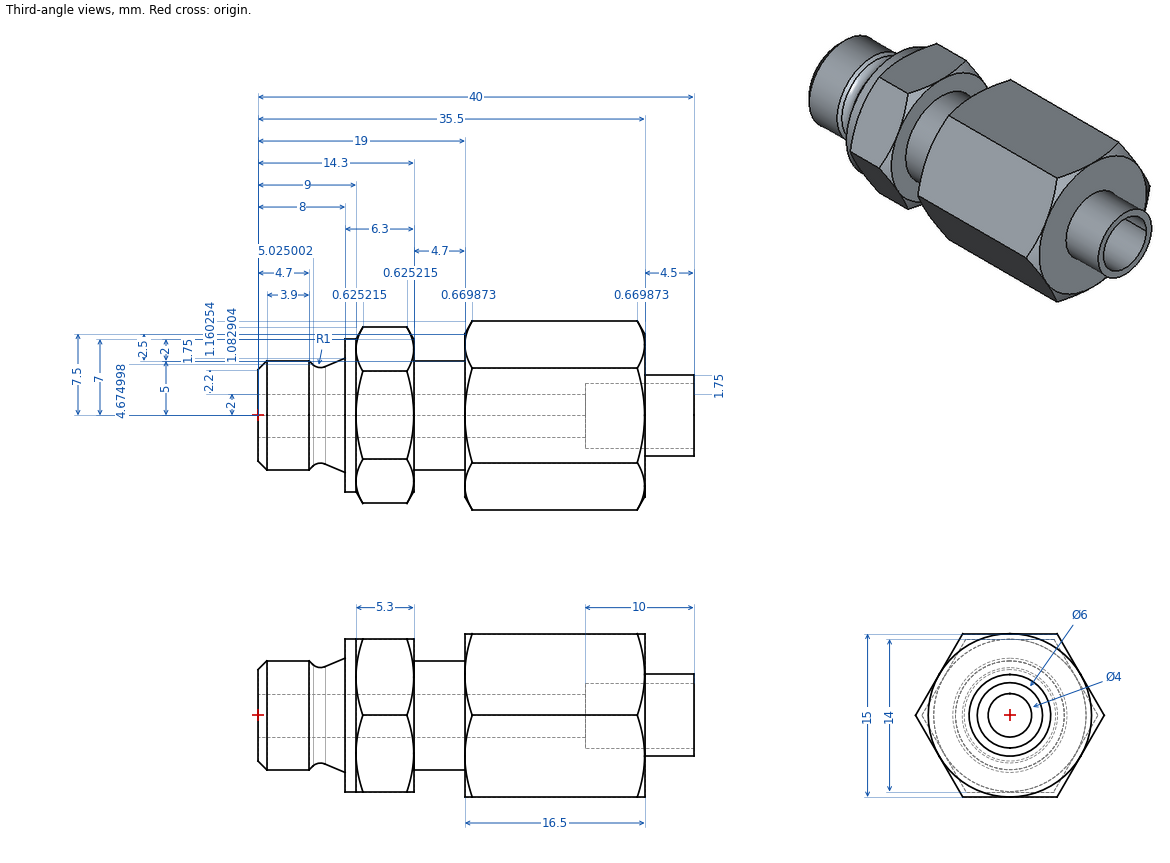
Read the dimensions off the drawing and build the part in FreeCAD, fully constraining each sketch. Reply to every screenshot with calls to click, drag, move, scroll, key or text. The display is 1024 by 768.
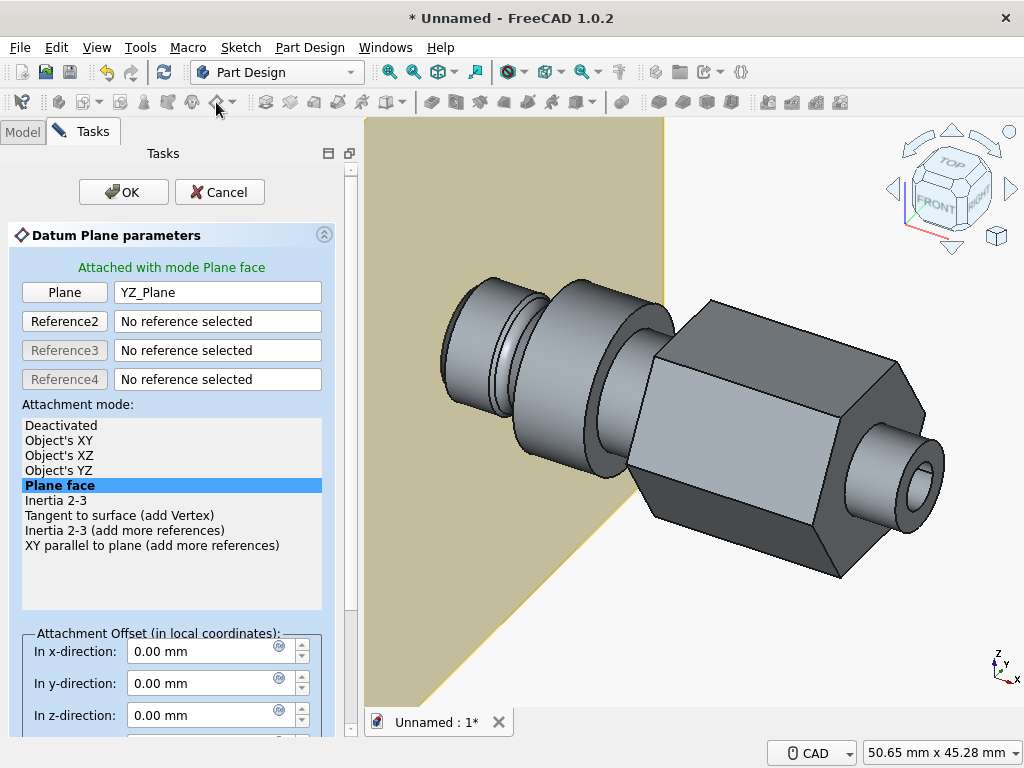
triple_click(210, 715)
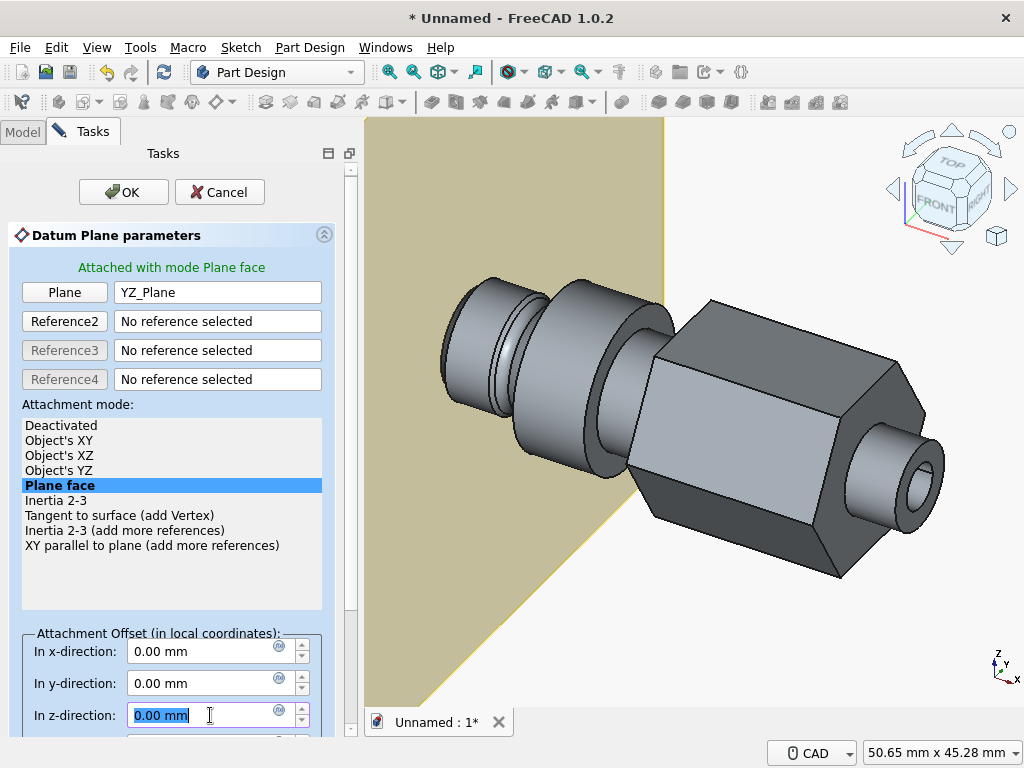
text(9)
key(Tab)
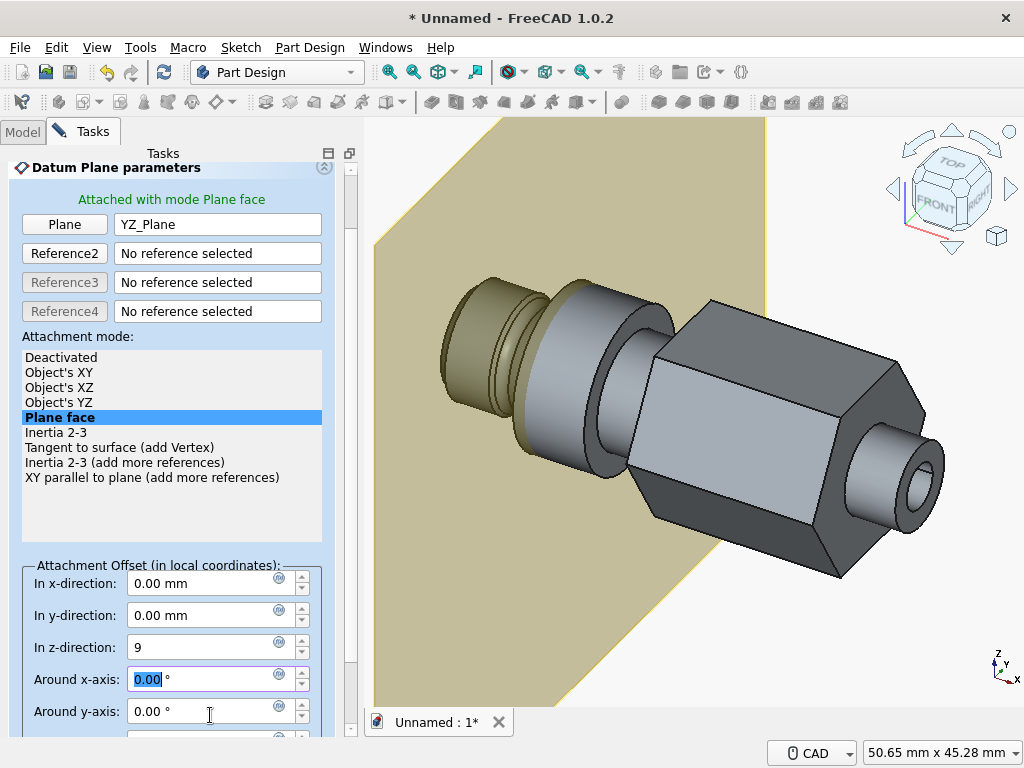
scroll(351, 450, up, 2)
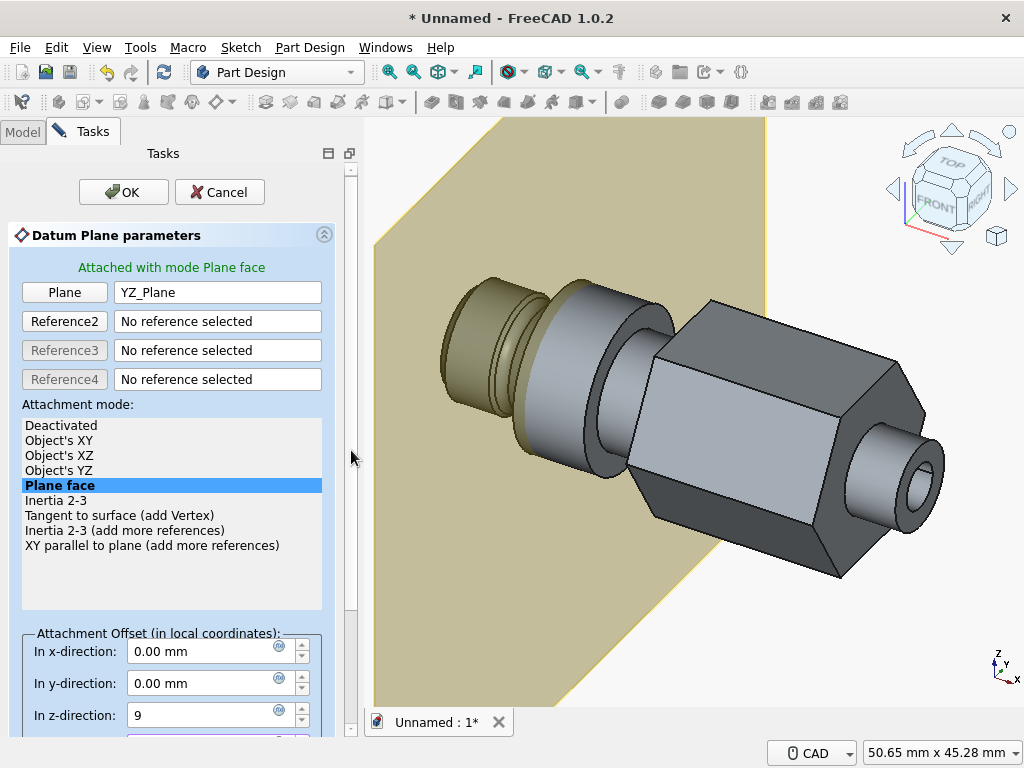
click(124, 192)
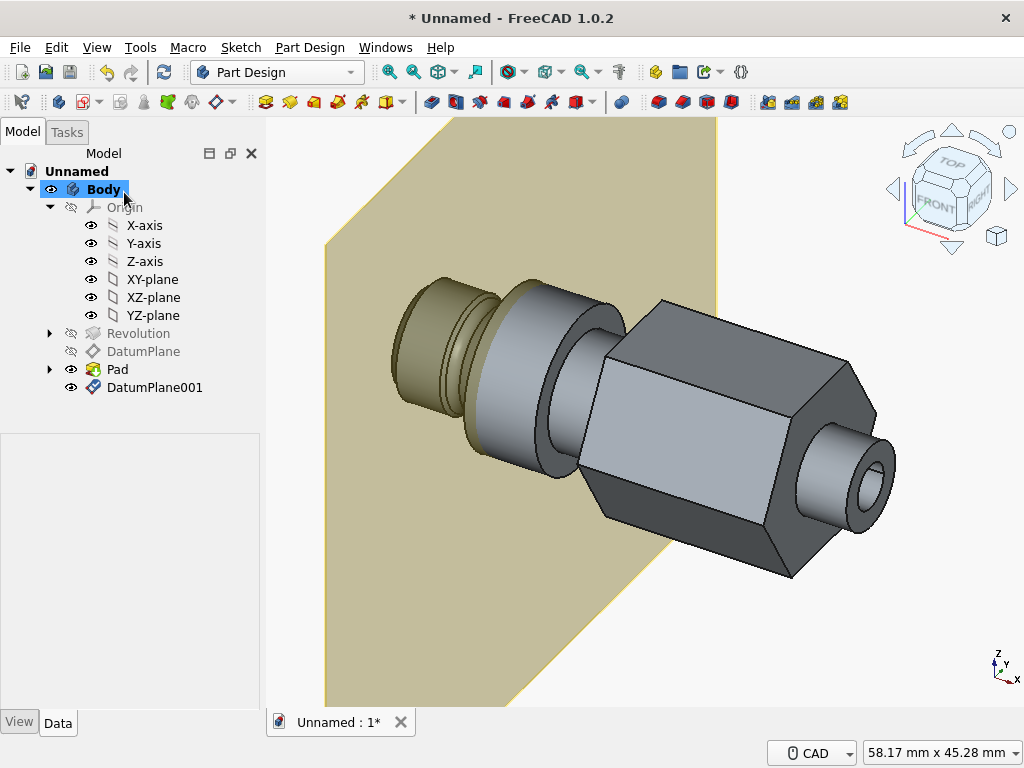
click(116, 387)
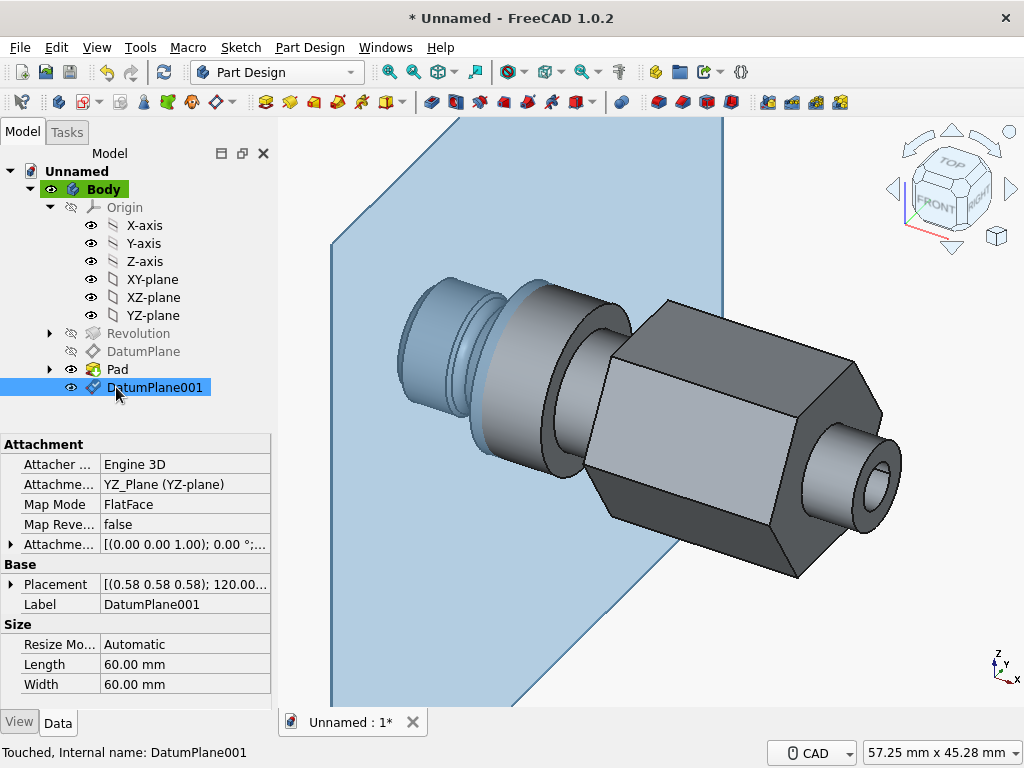
click(84, 102)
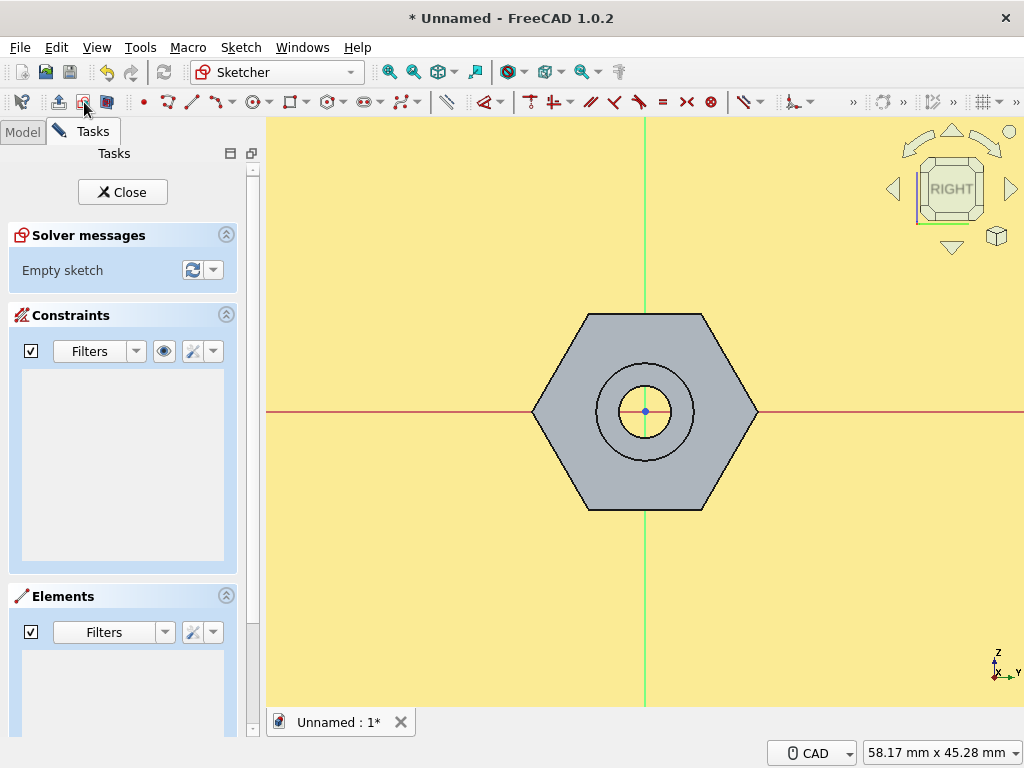
key(q)
key(s)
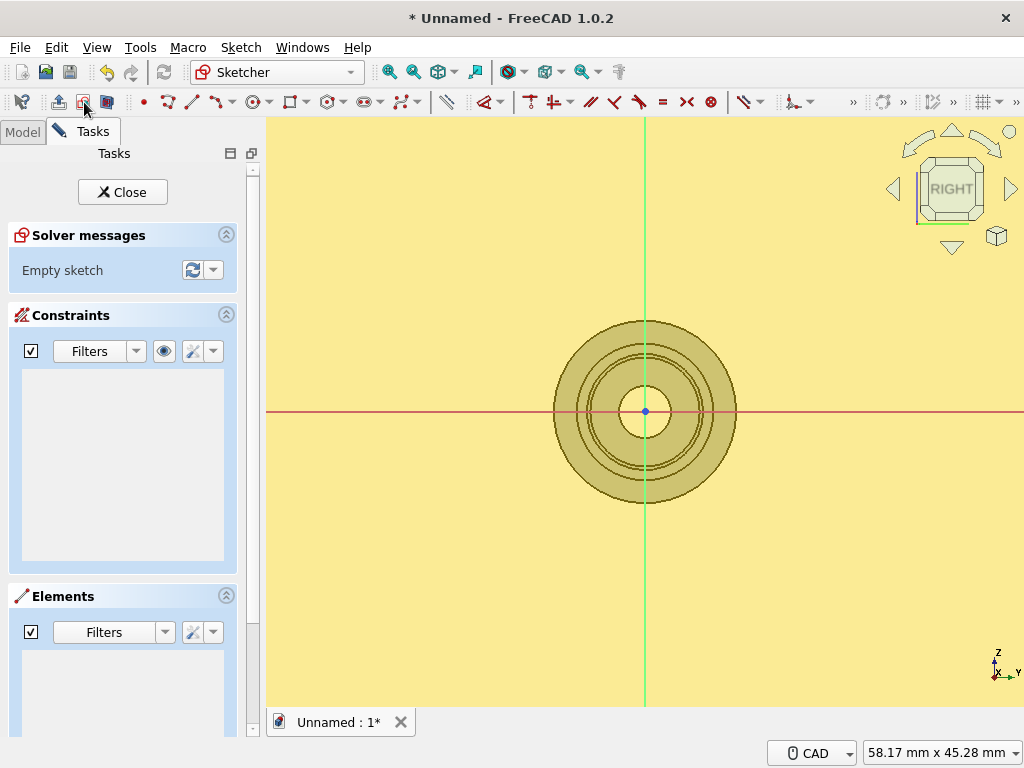
scroll(728, 412, up, 3)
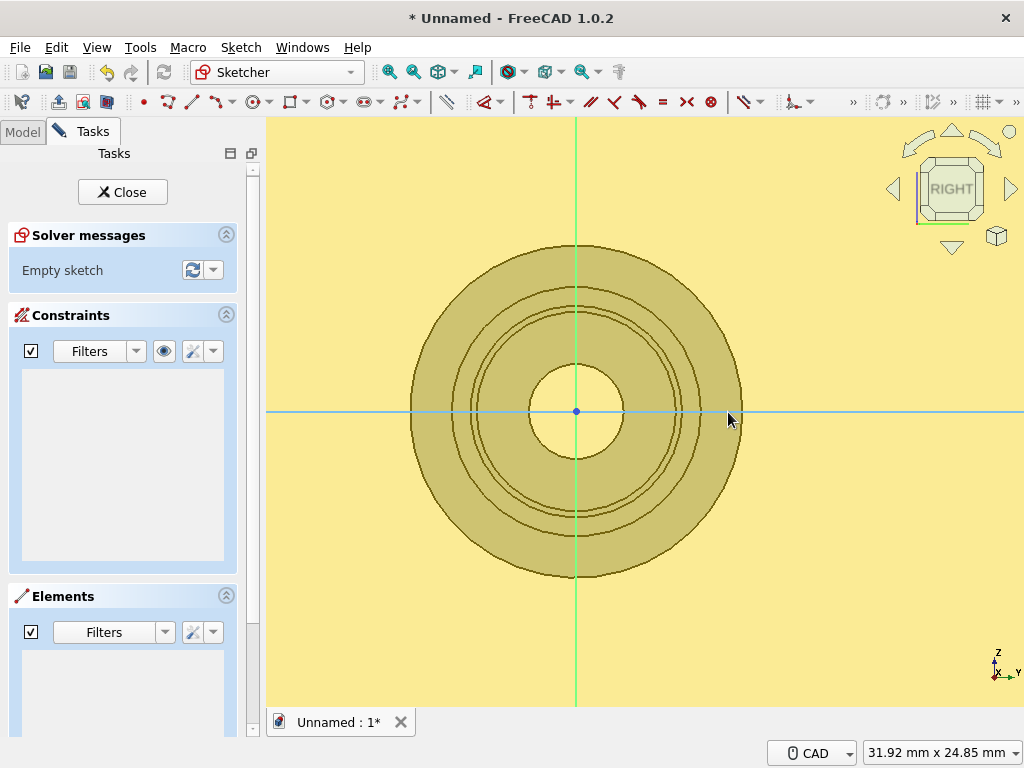
key(g)
key(p)
key(6)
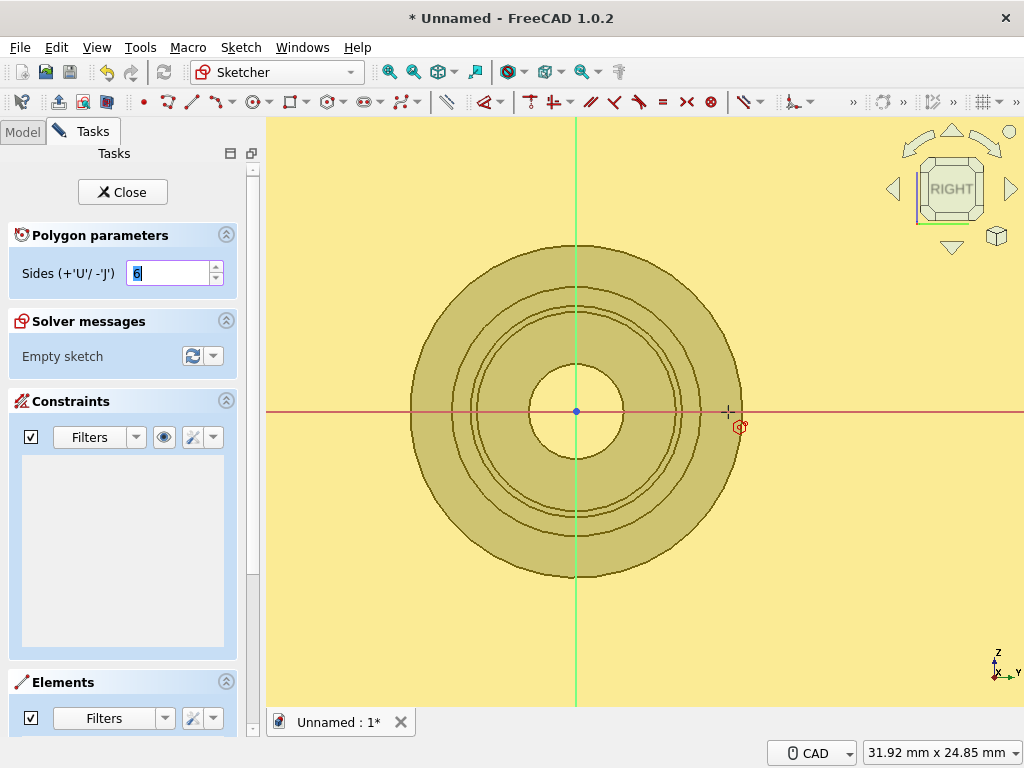
click(576, 412)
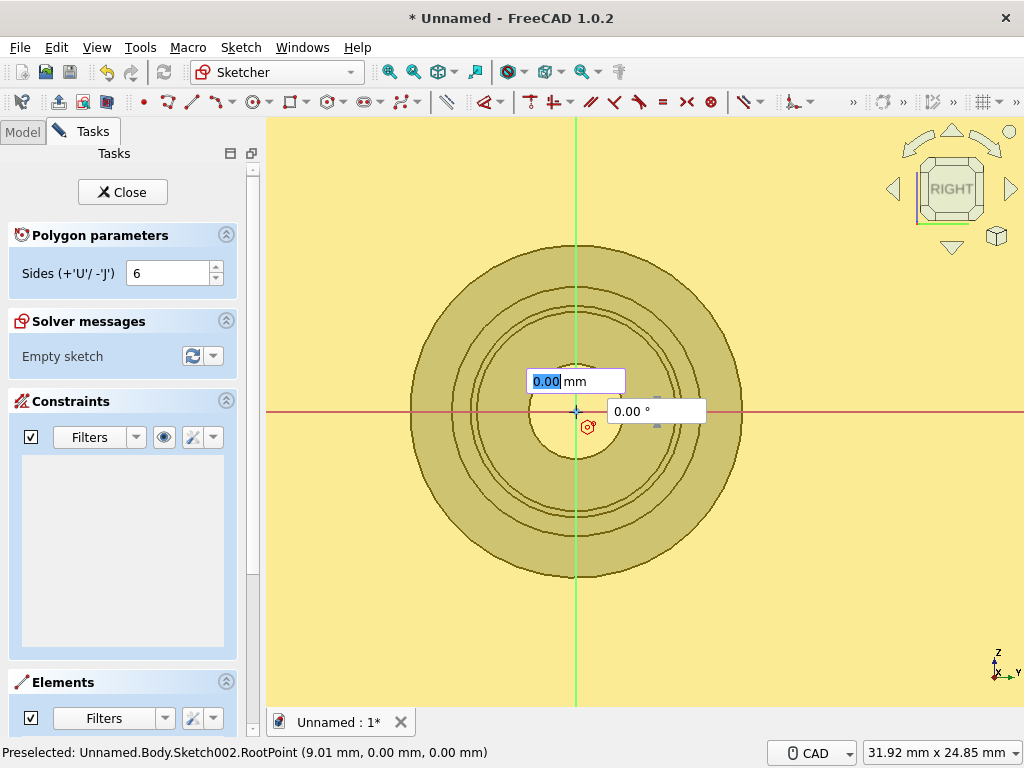
click(384, 412)
right_click(384, 412)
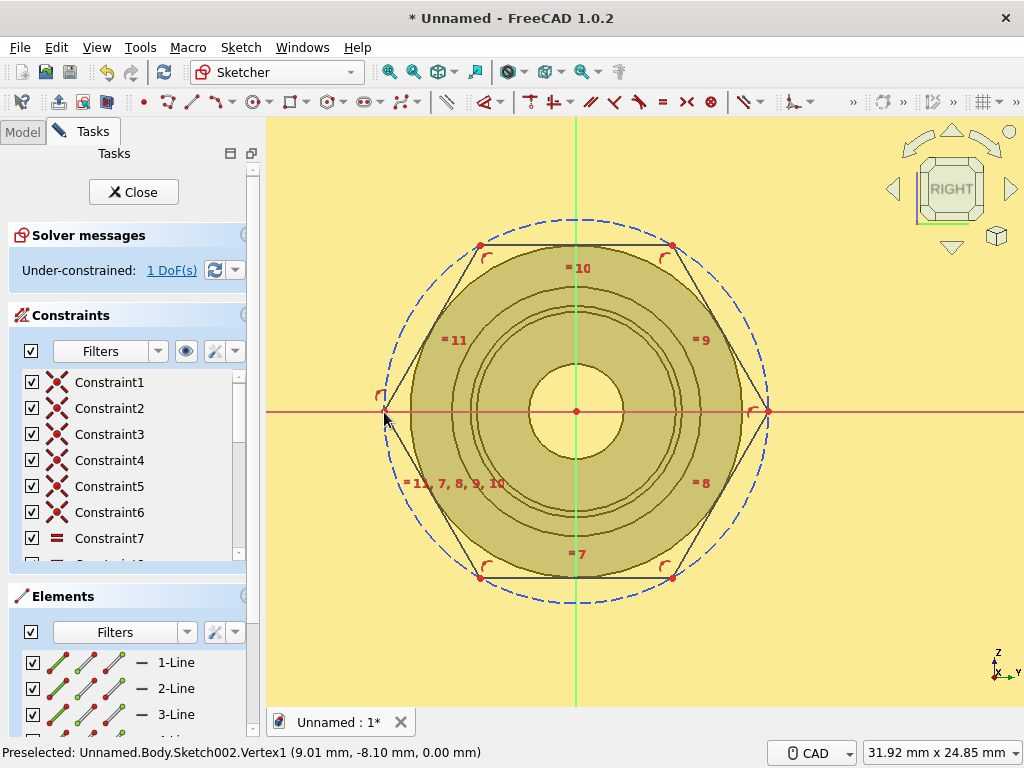
key(g)
key(c)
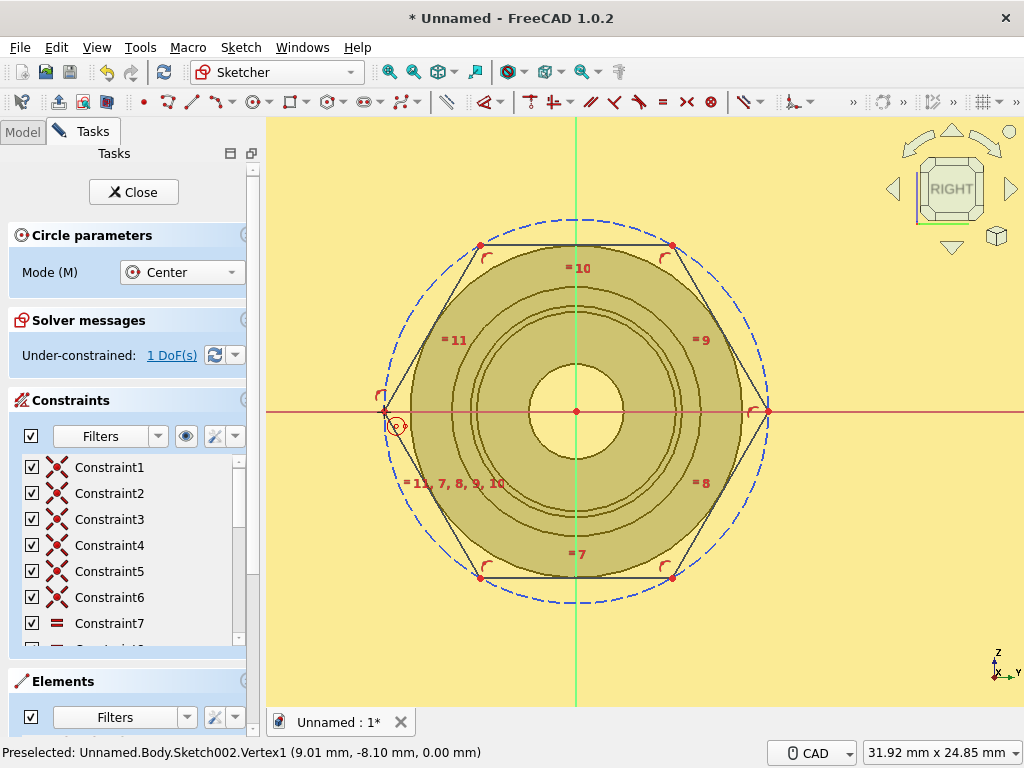
click(576, 412)
click(610, 378)
key(Escape)